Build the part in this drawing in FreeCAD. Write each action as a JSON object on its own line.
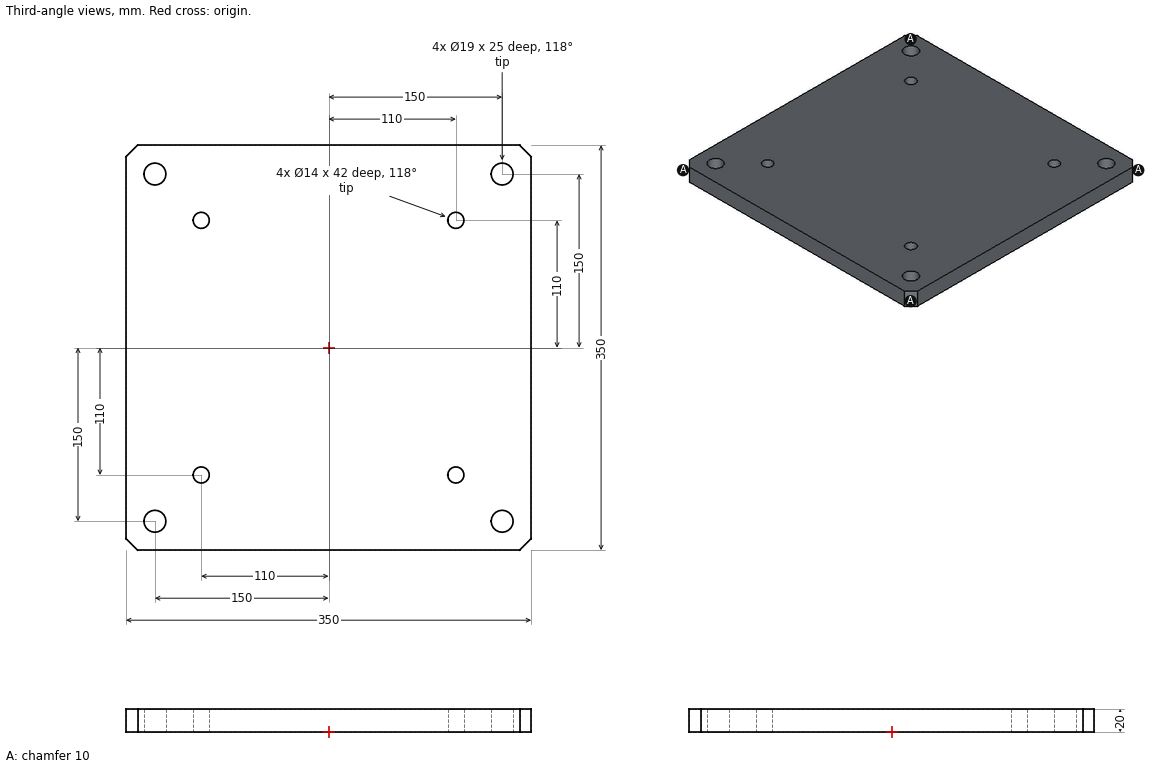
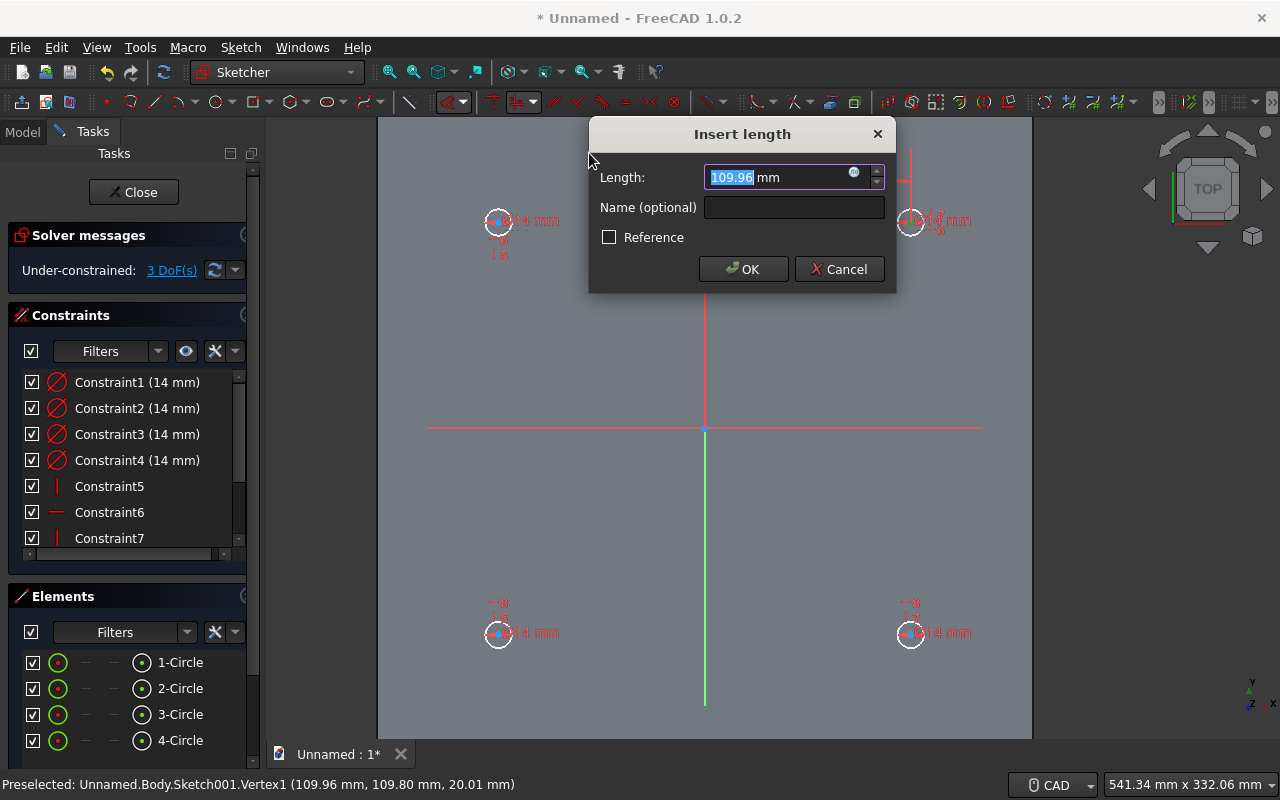
{"action": "type", "text": "110"}
{"action": "key", "text": "Return"}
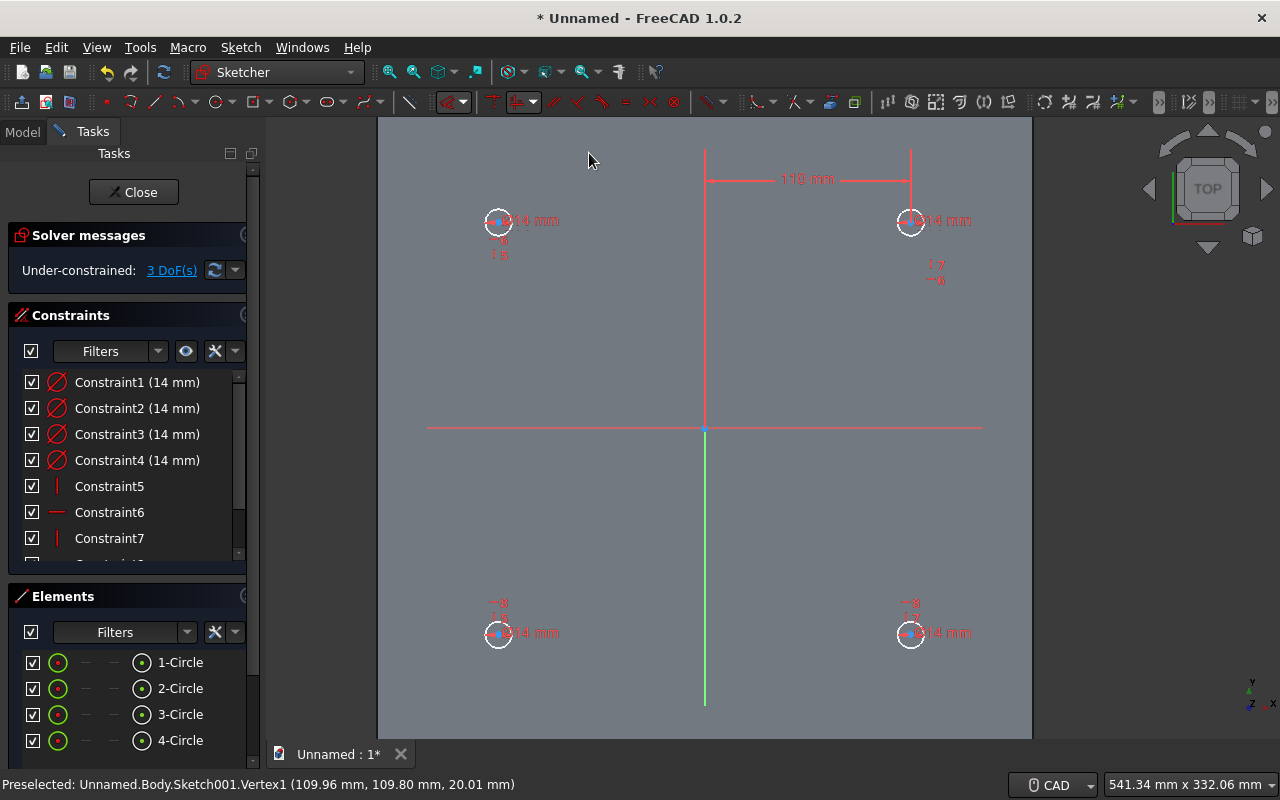
{"action": "left_click", "coordinate": [911, 223]}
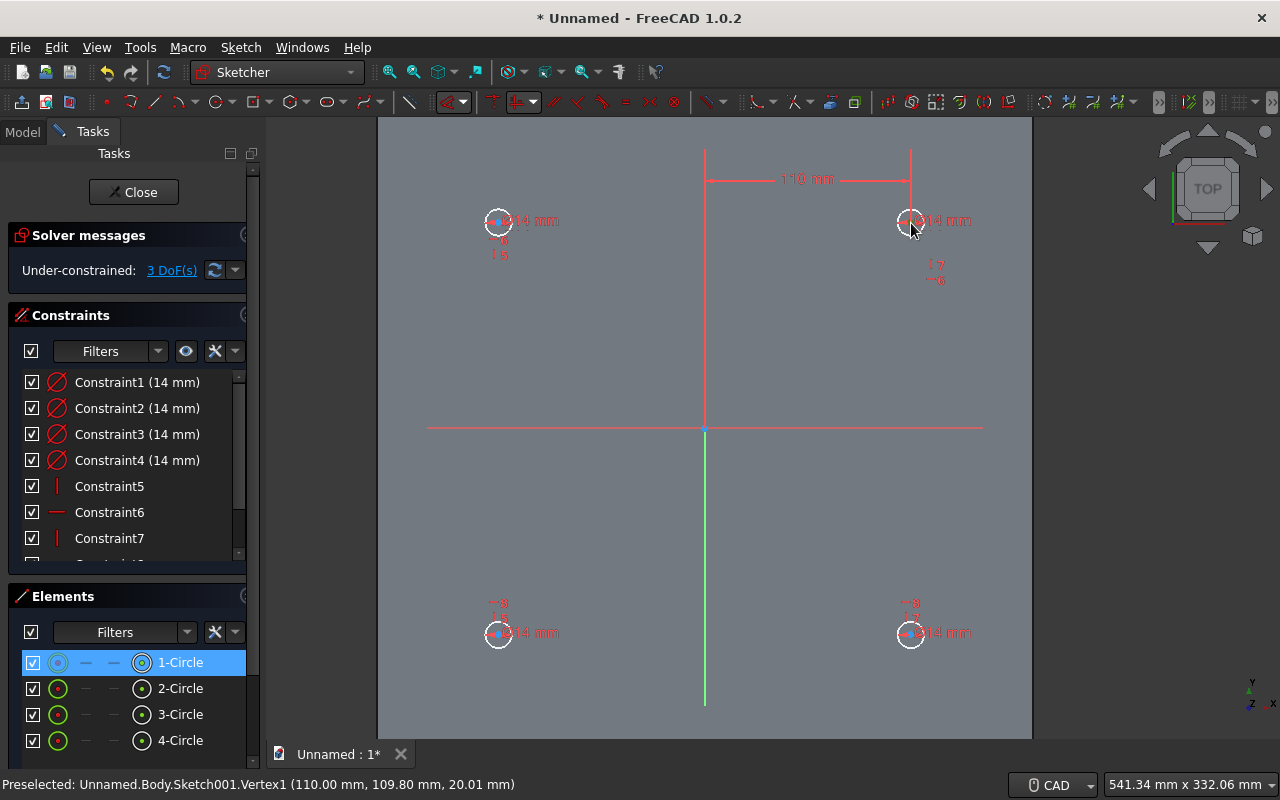
{"action": "key", "text": "i"}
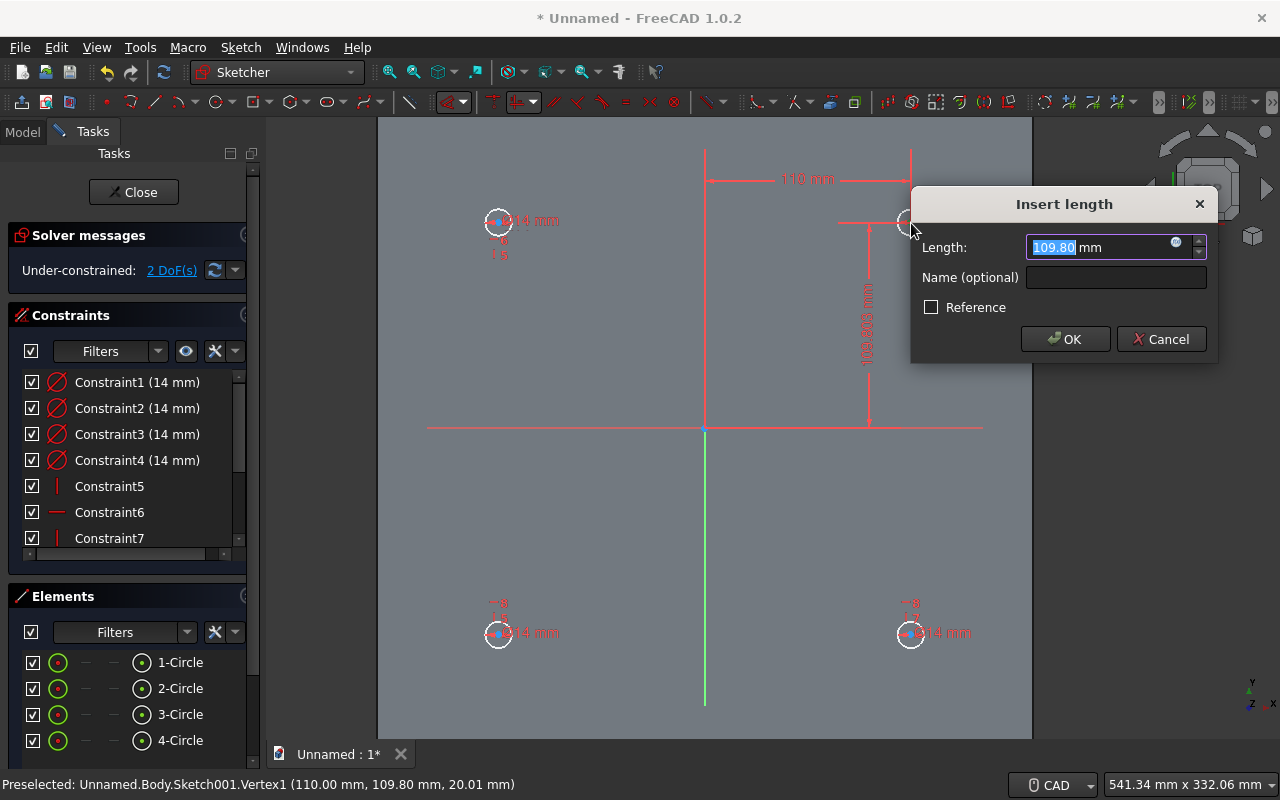
{"action": "type", "text": "110"}
{"action": "key", "text": "Return"}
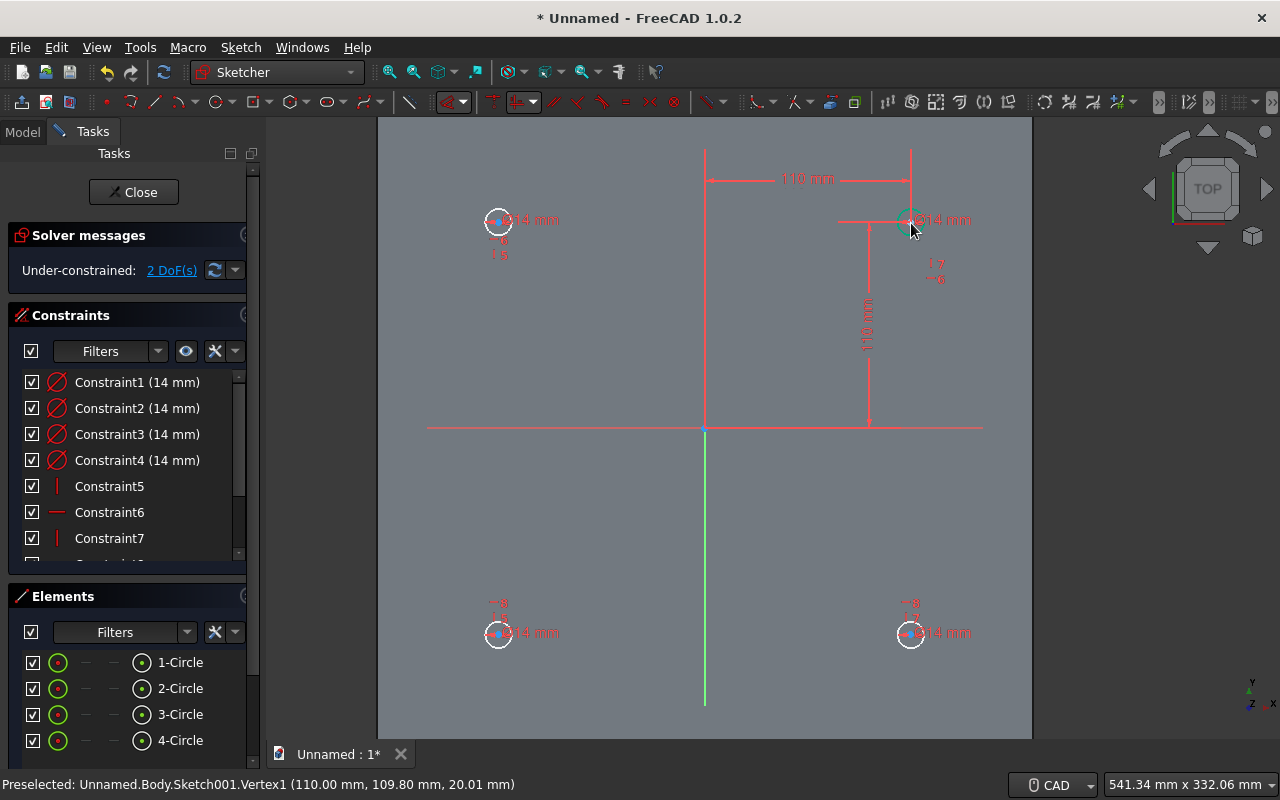
{"action": "left_click", "coordinate": [499, 635]}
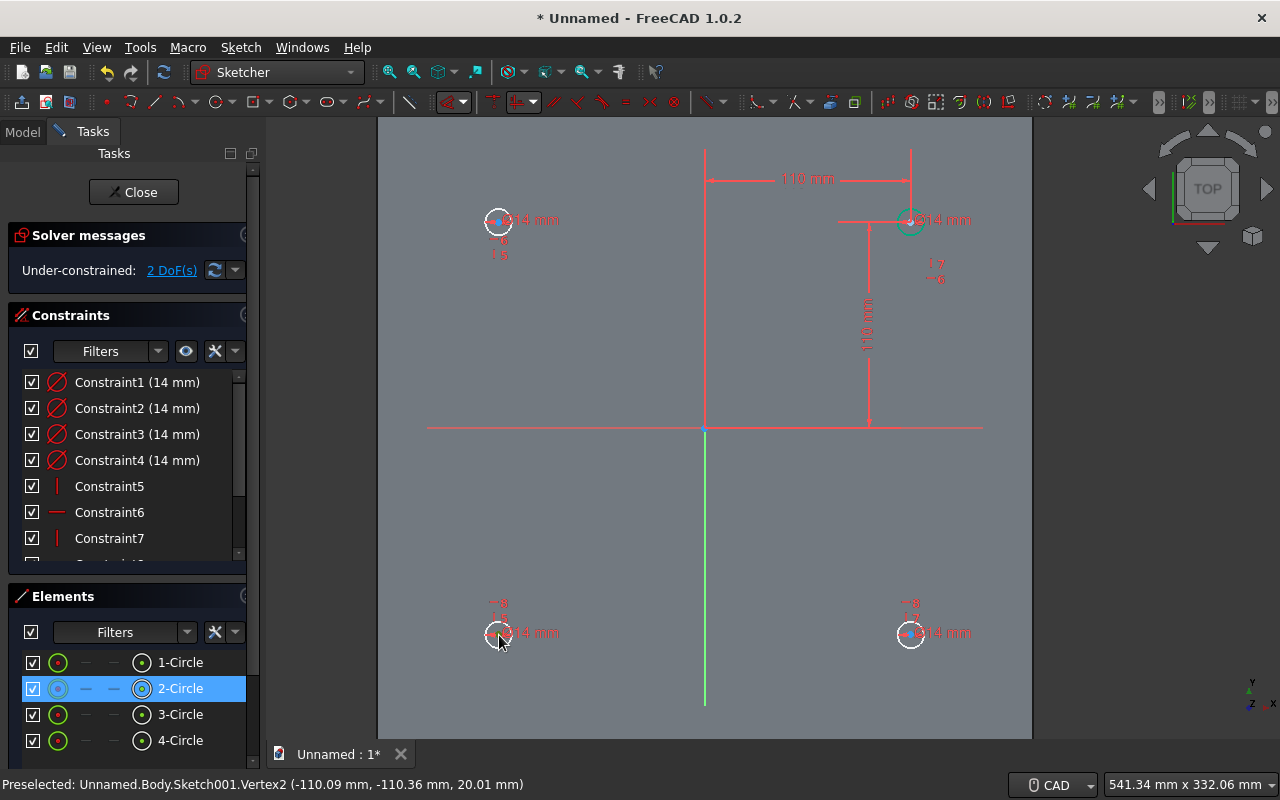
{"action": "key", "text": "l"}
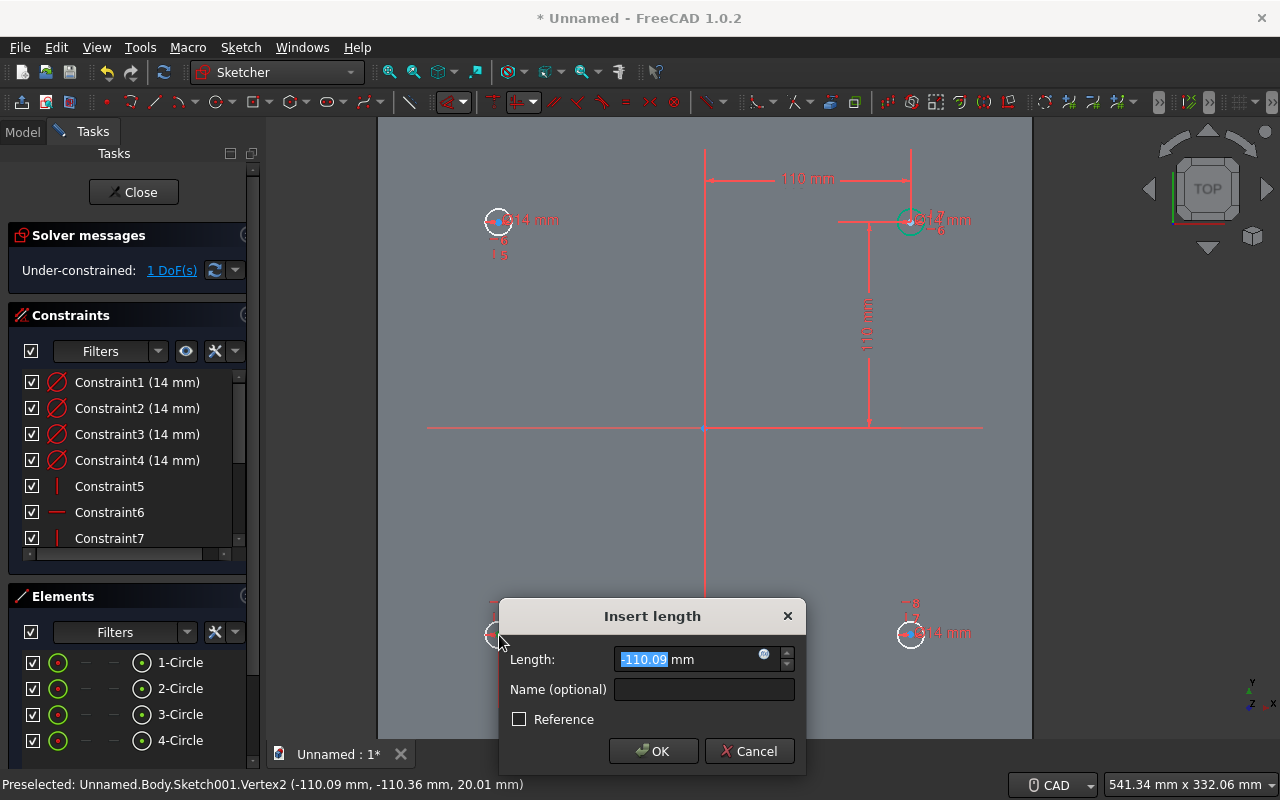
{"action": "type", "text": "-110"}
{"action": "key", "text": "Return"}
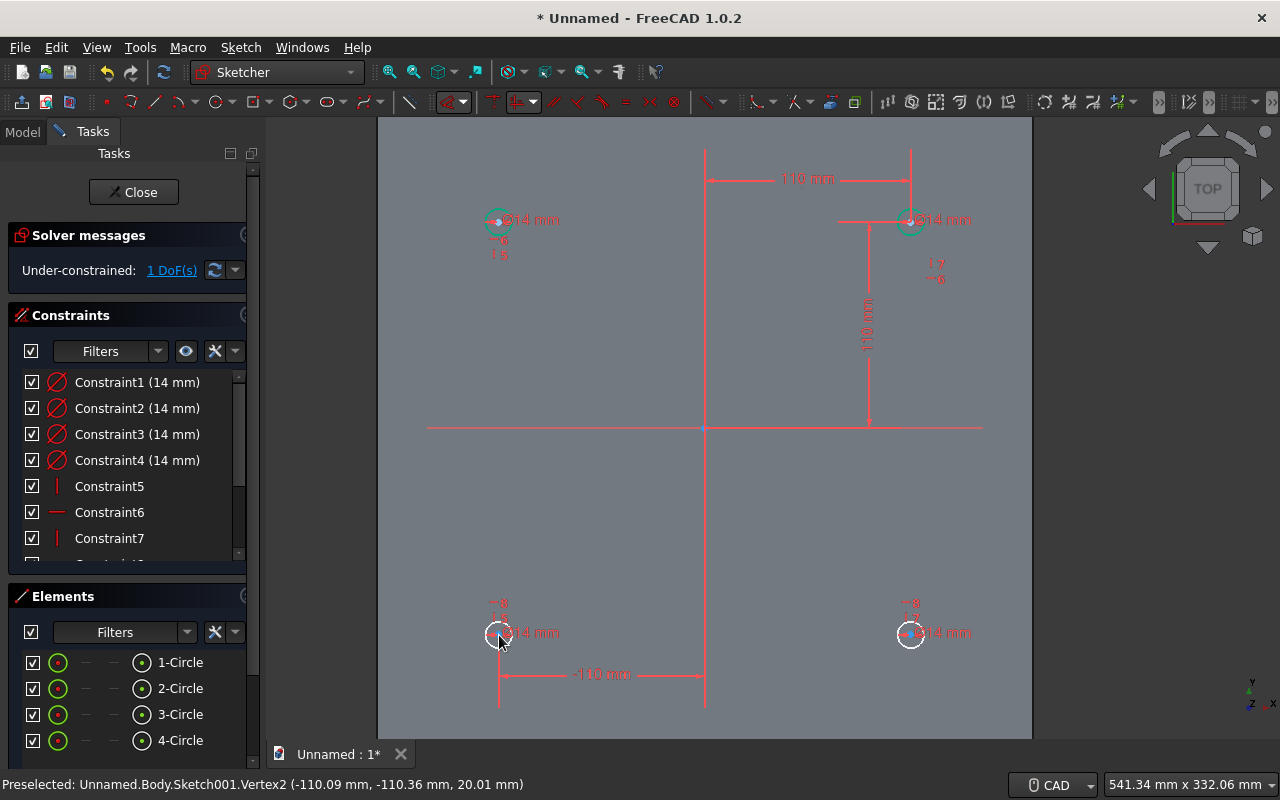
{"action": "left_click", "coordinate": [499, 635]}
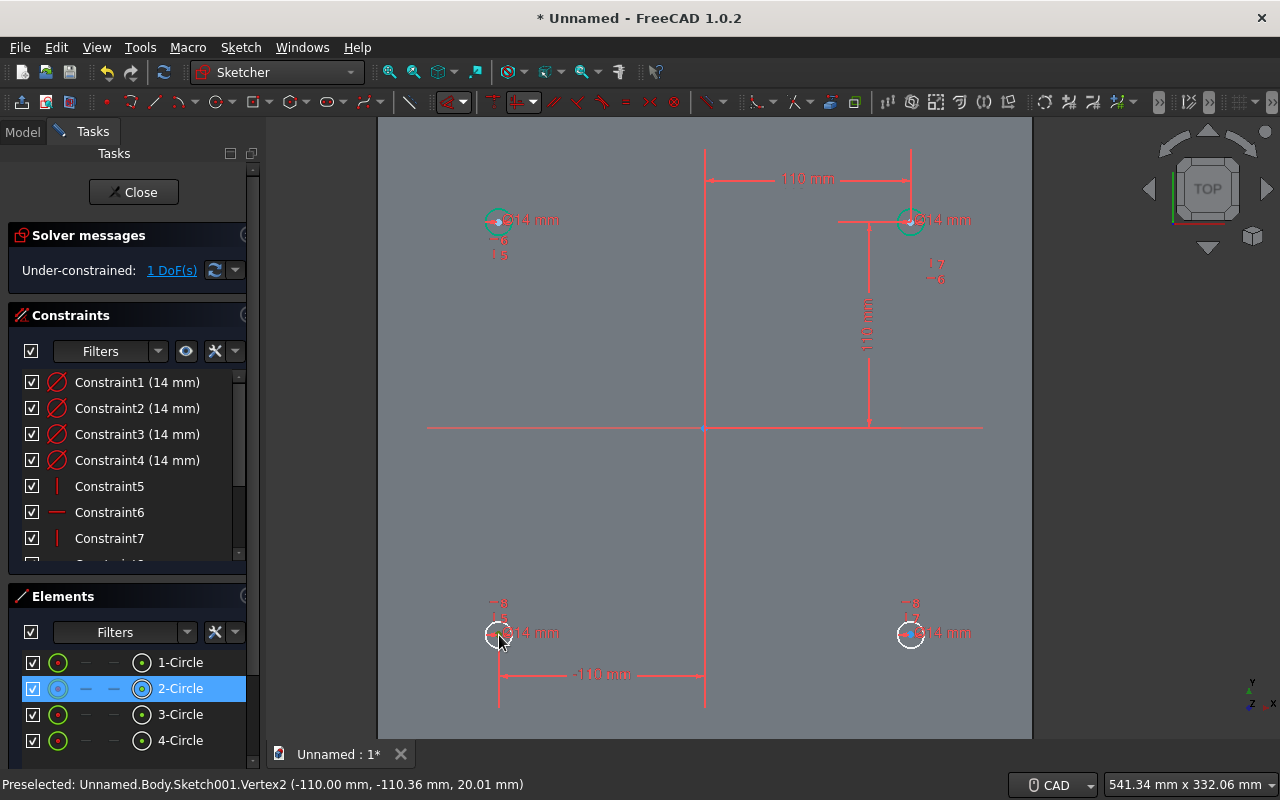
{"action": "left_click", "coordinate": [466, 102]}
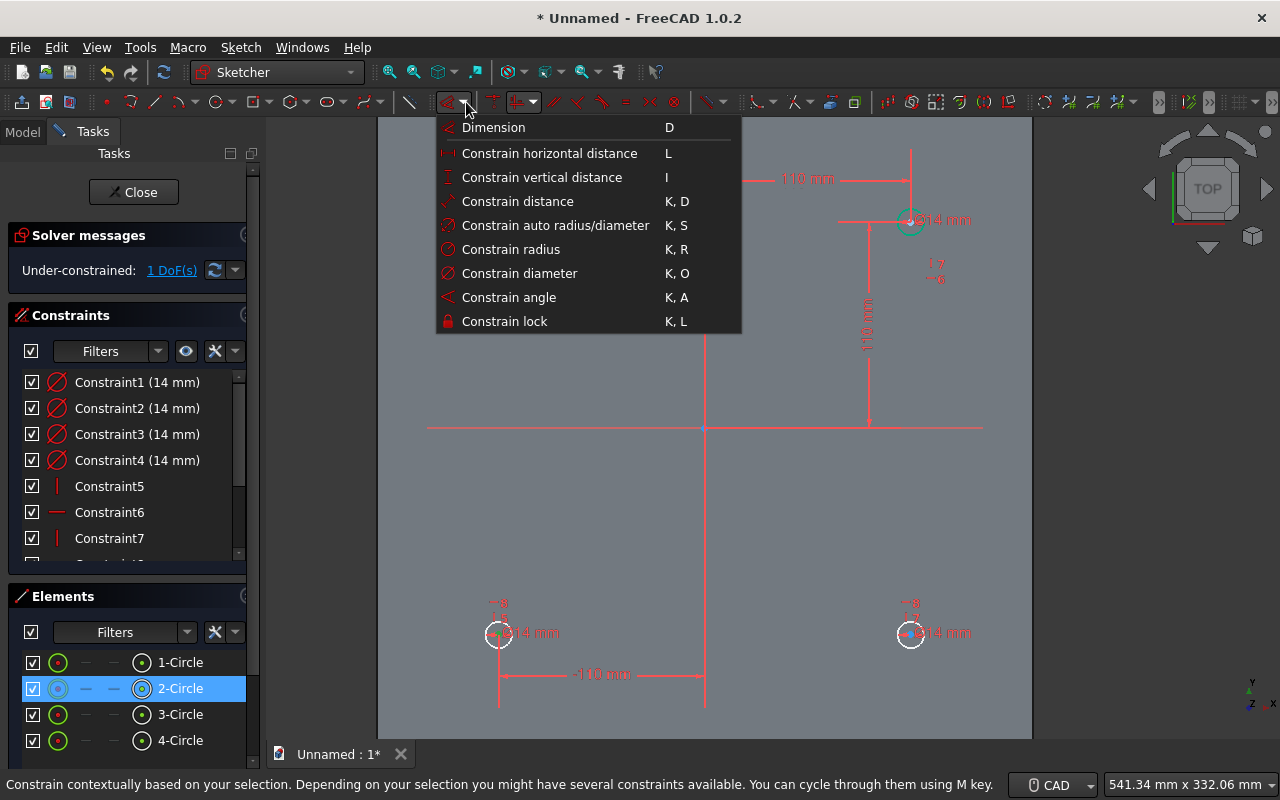
{"action": "left_click", "coordinate": [589, 177]}